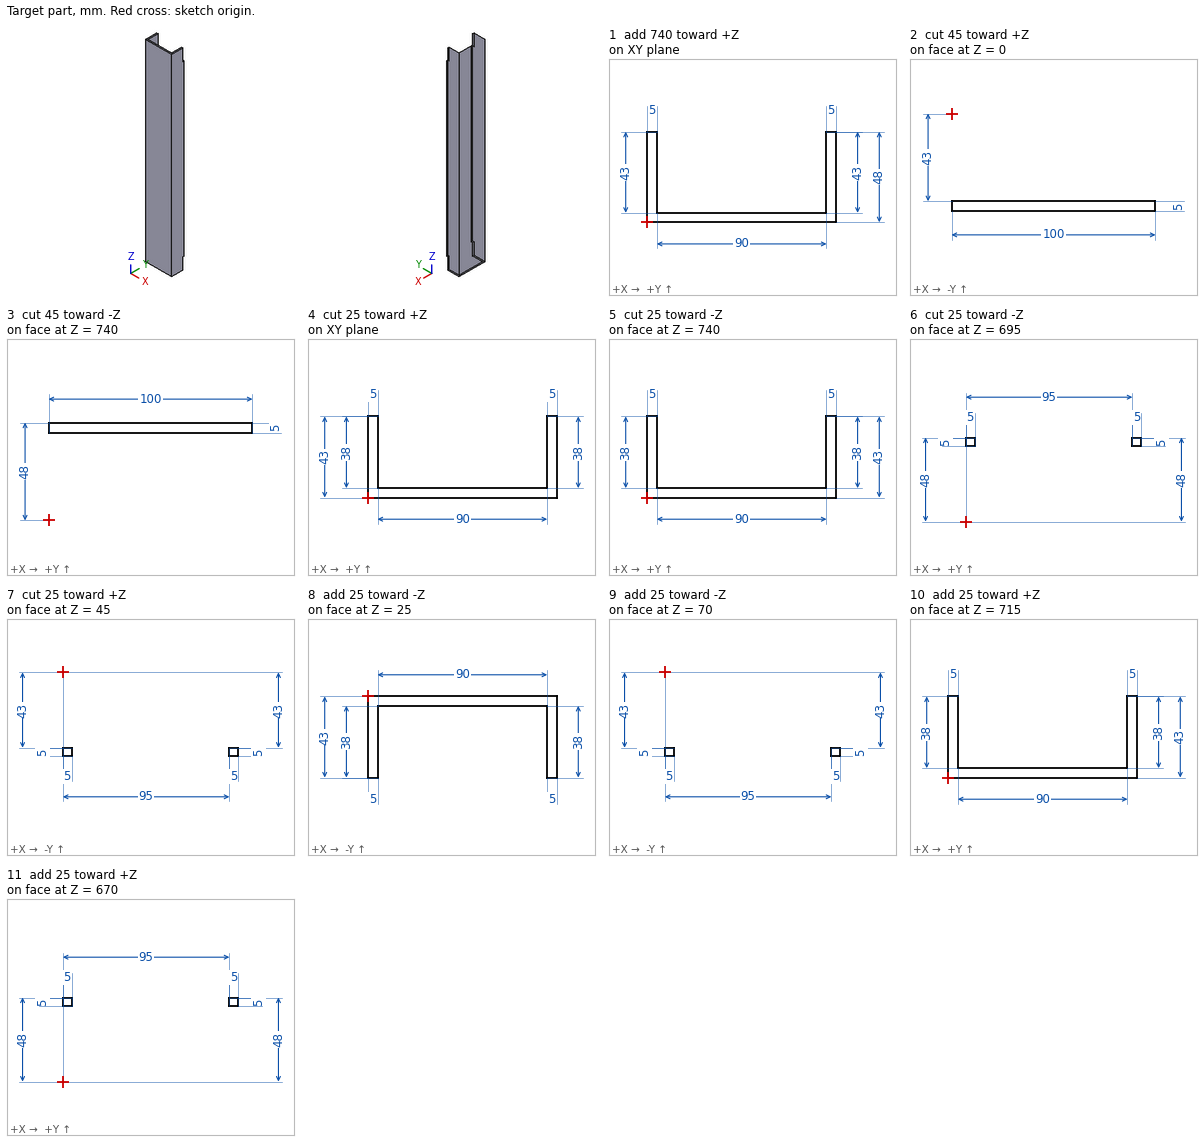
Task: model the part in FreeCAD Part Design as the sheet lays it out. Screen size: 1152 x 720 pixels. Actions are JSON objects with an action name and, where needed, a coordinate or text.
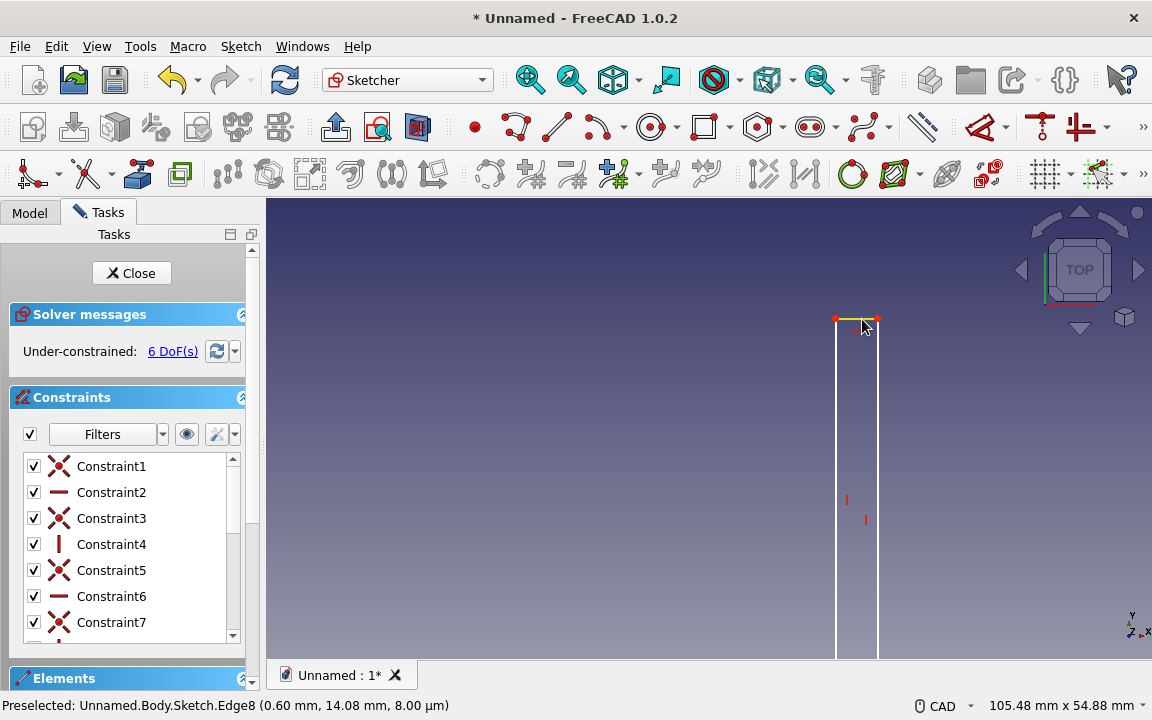
{"action": "left_click", "coordinate": [861, 319]}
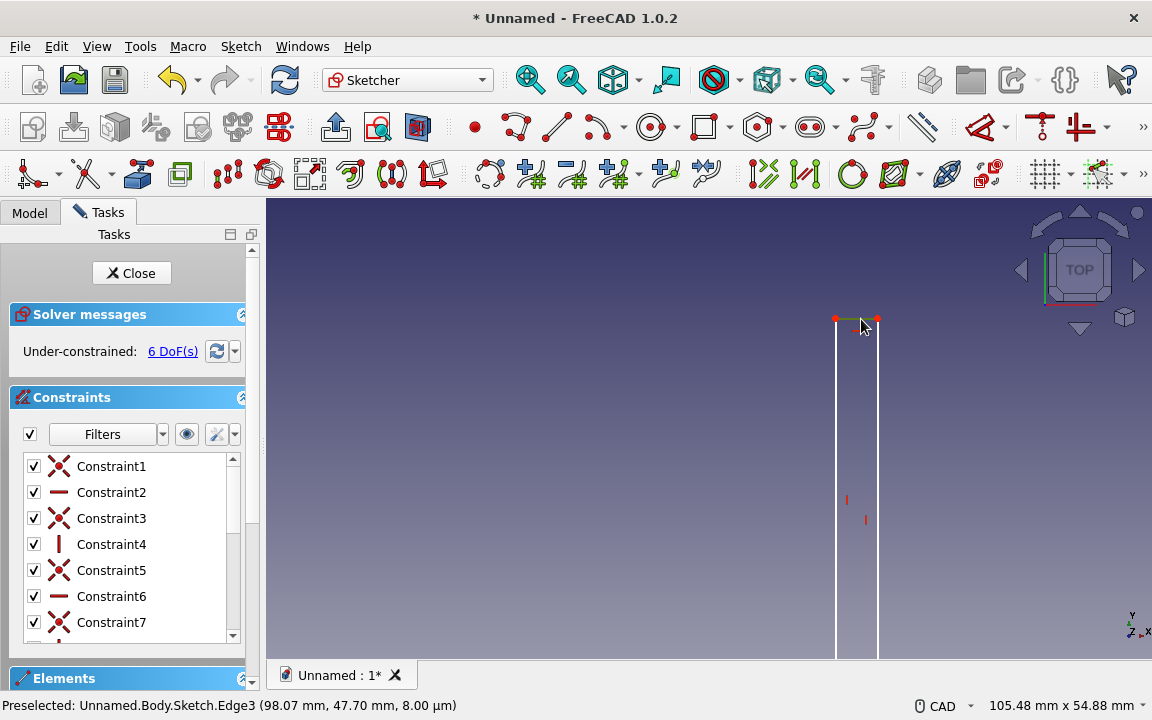
{"action": "left_click", "coordinate": [1006, 128]}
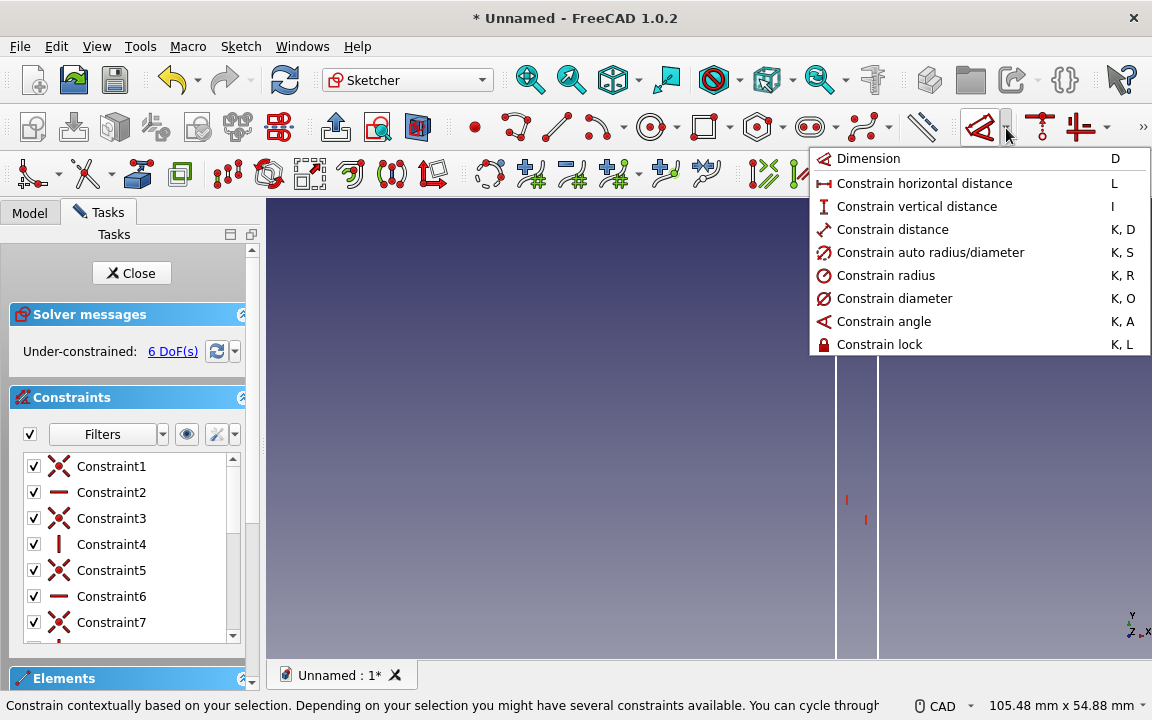
{"action": "left_click", "coordinate": [980, 184]}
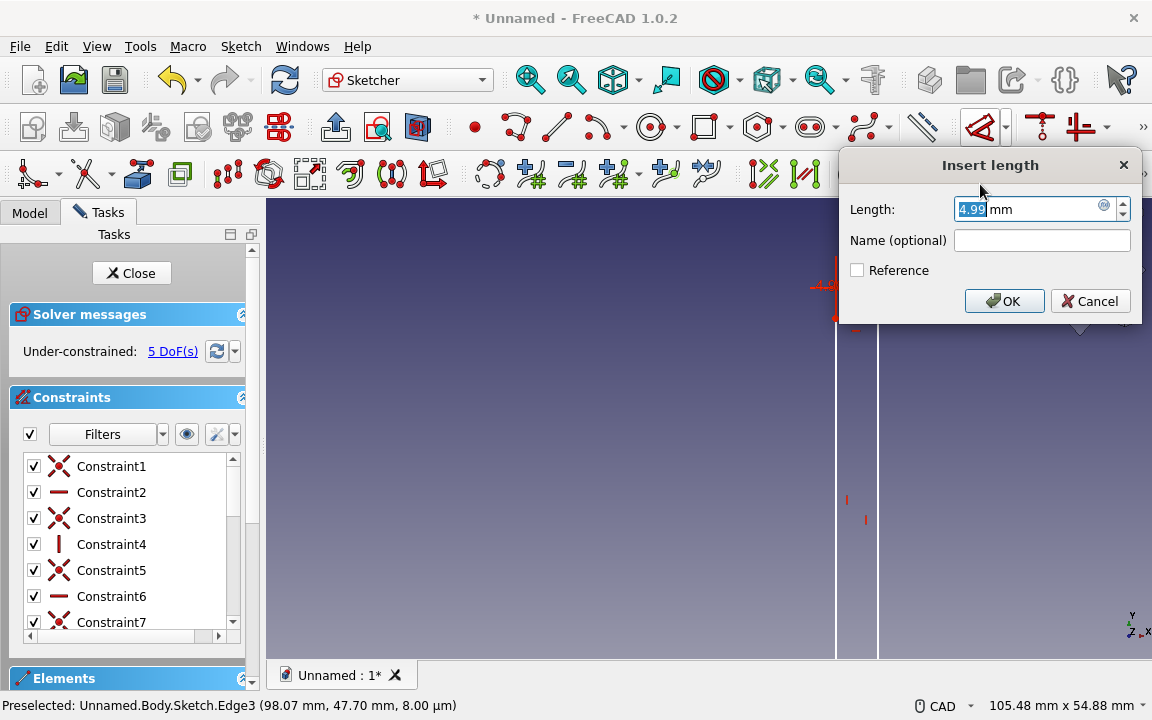
{"action": "type", "text": "5"}
{"action": "key", "text": "Return"}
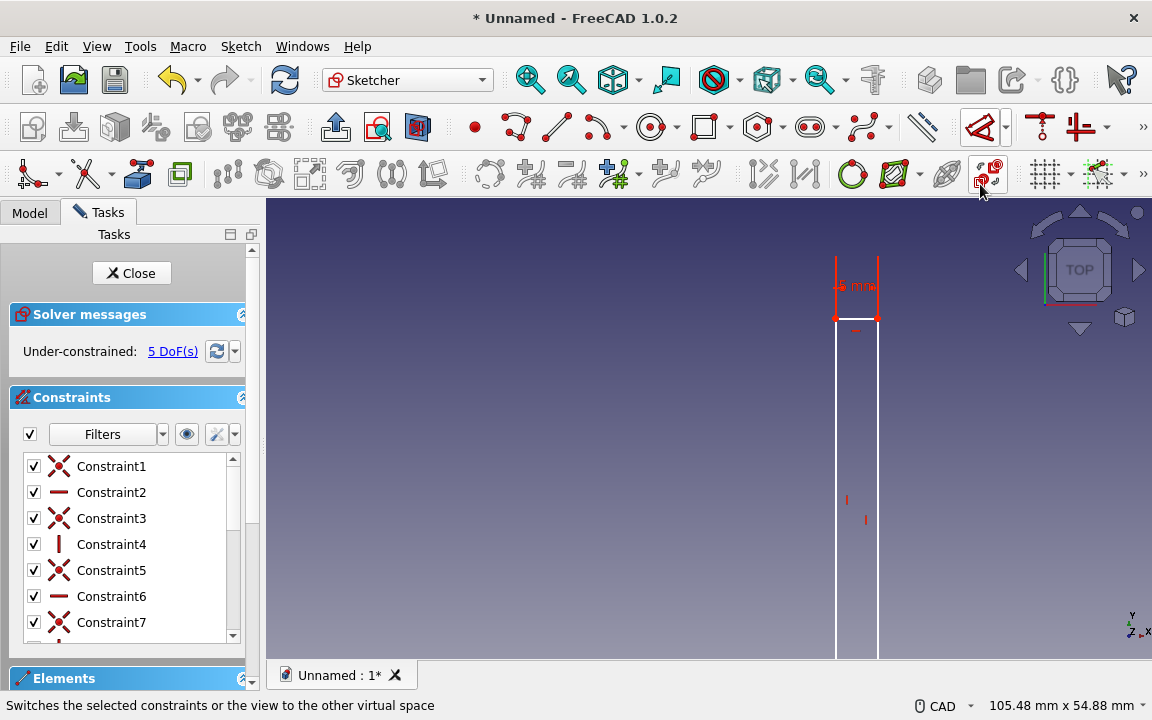
{"action": "scroll", "coordinate": [863, 320], "scroll_direction": "down", "scroll_amount": 3}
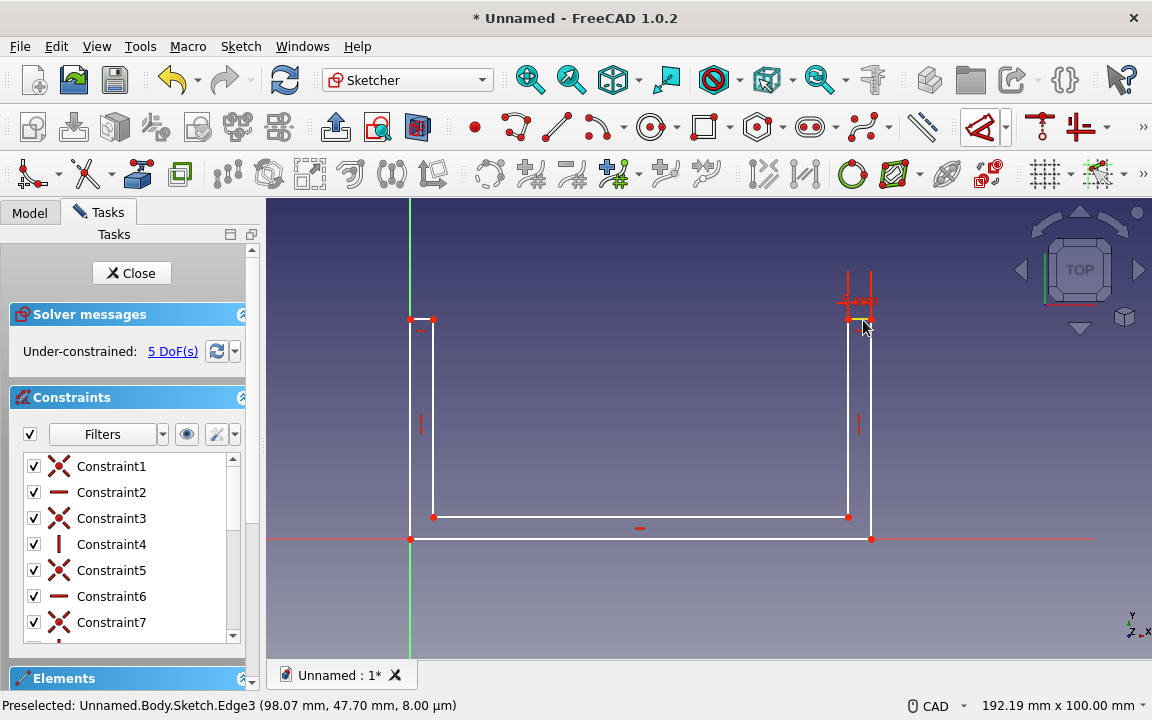
{"action": "scroll", "coordinate": [426, 319], "scroll_direction": "up", "scroll_amount": 4}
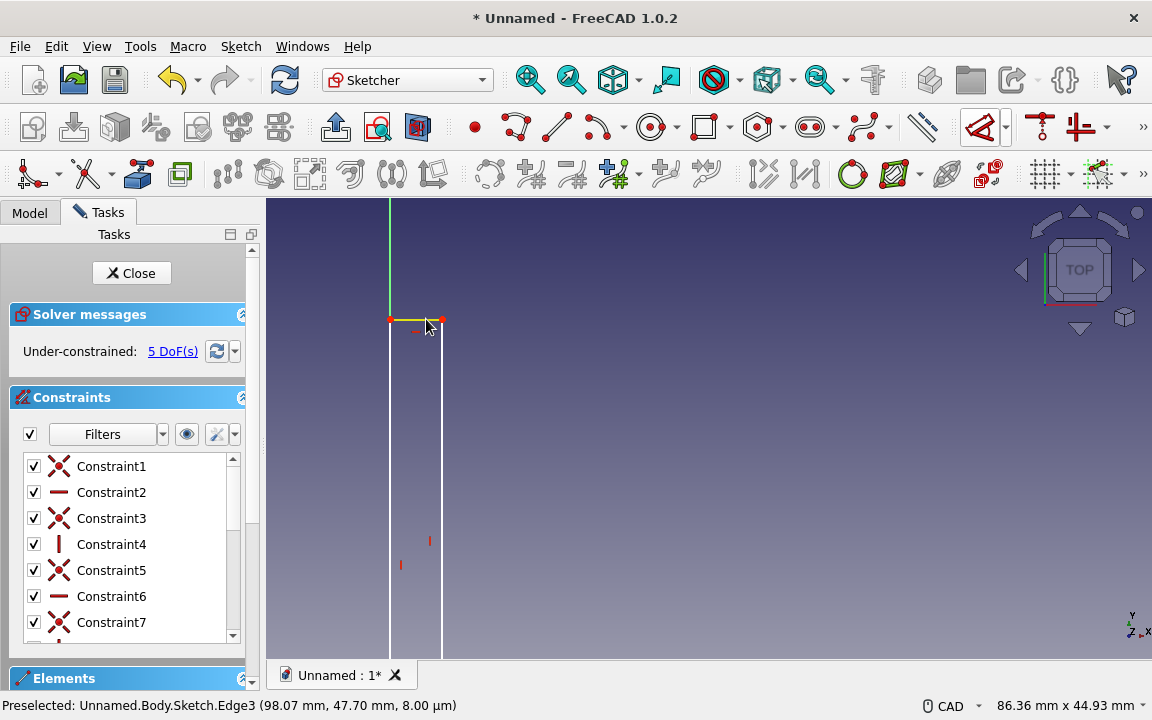
{"action": "left_click", "coordinate": [427, 320]}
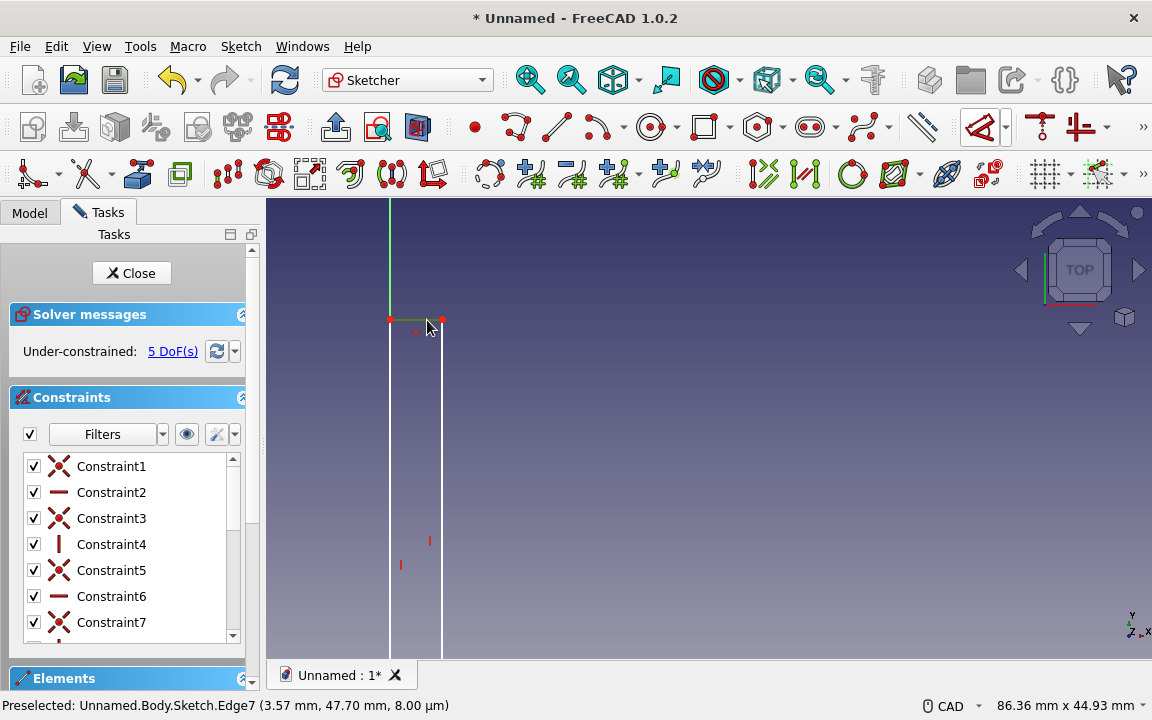
{"action": "key", "text": "l"}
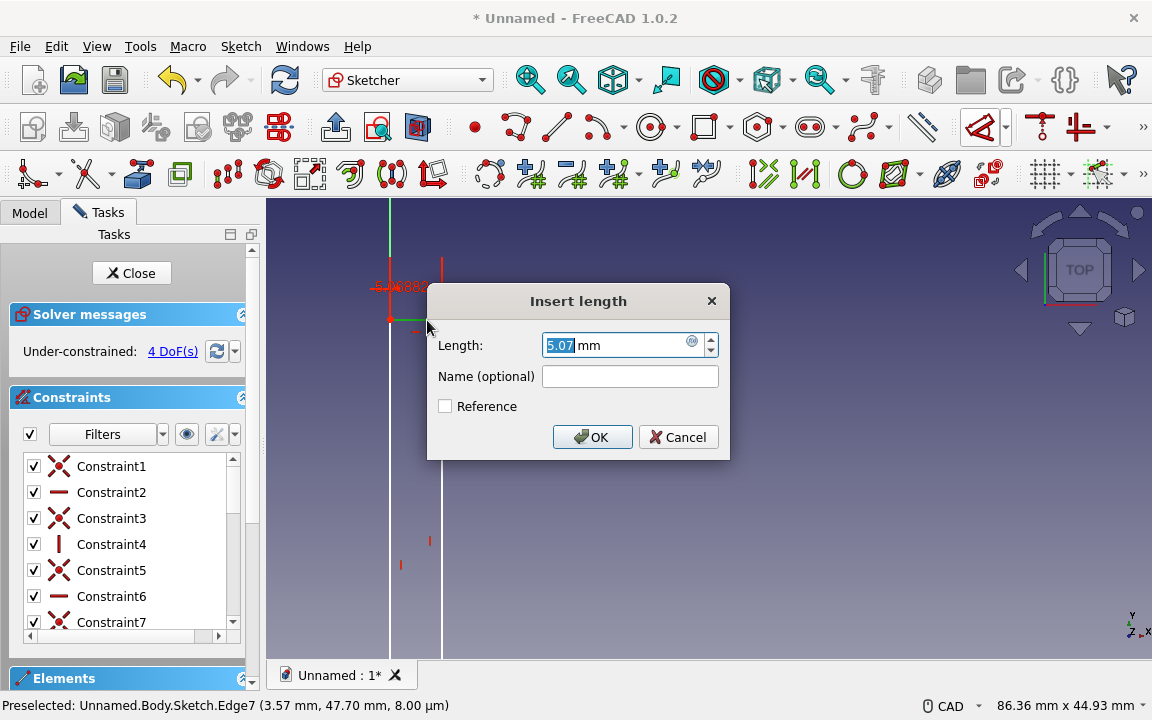
{"action": "type", "text": "5"}
{"action": "key", "text": "Return"}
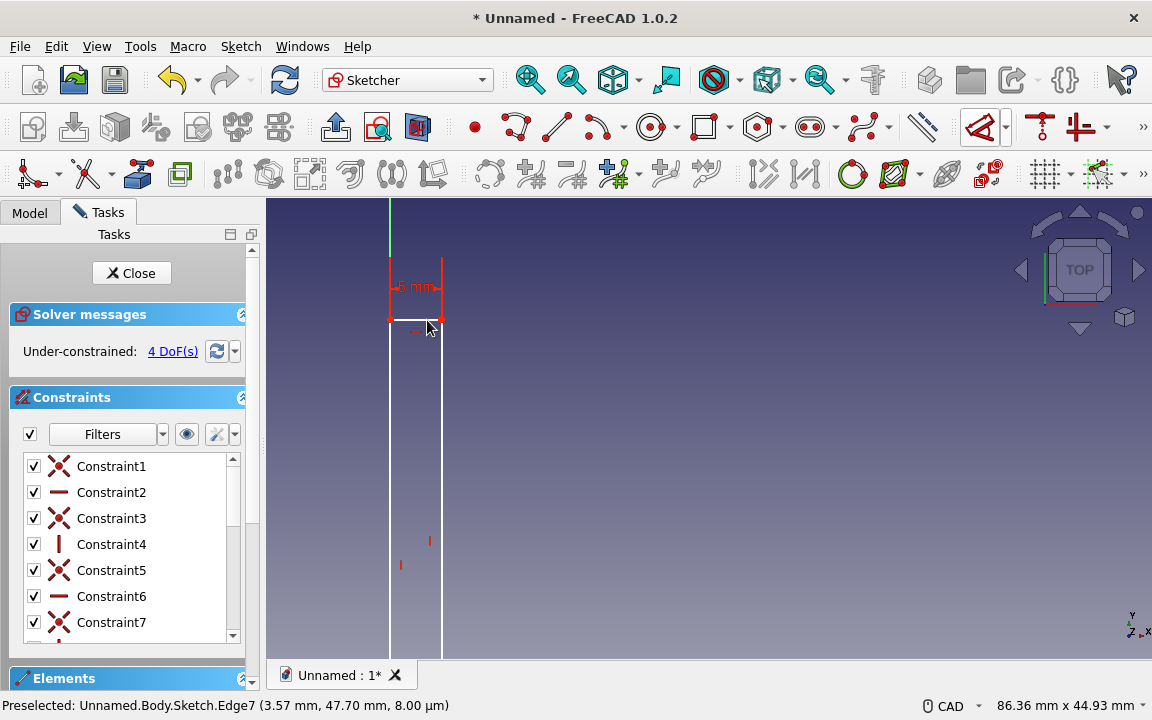
{"action": "scroll", "coordinate": [426, 319], "scroll_direction": "down", "scroll_amount": 4}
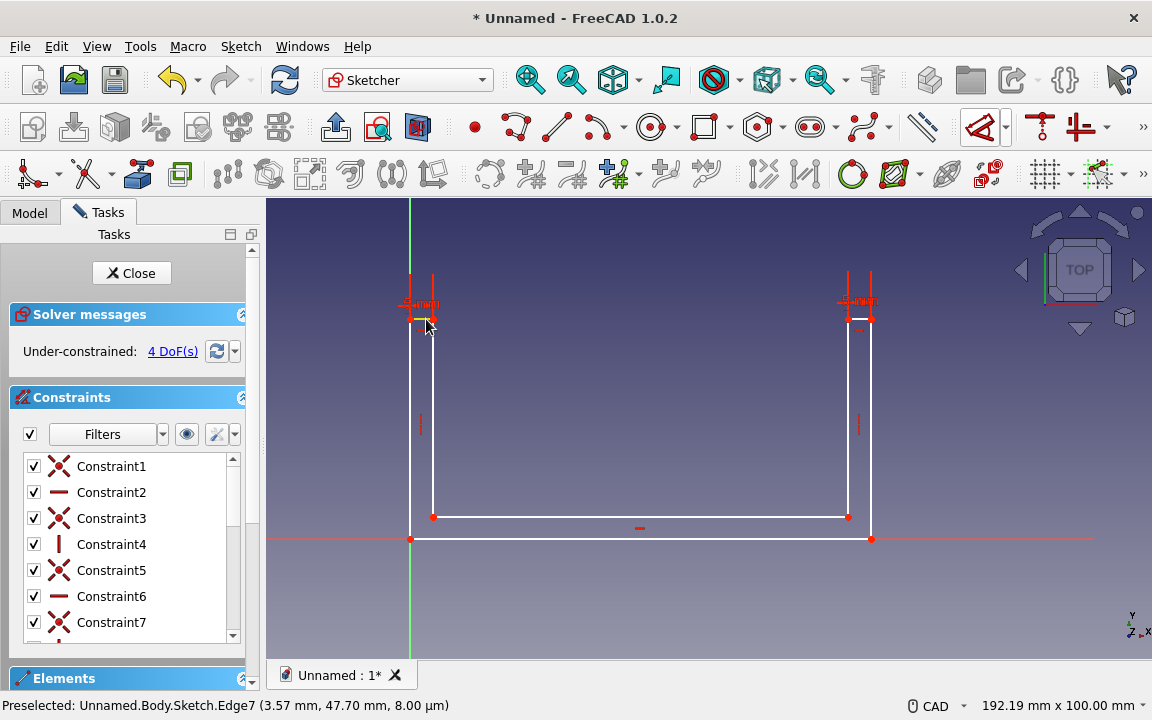
{"action": "left_click", "coordinate": [872, 473]}